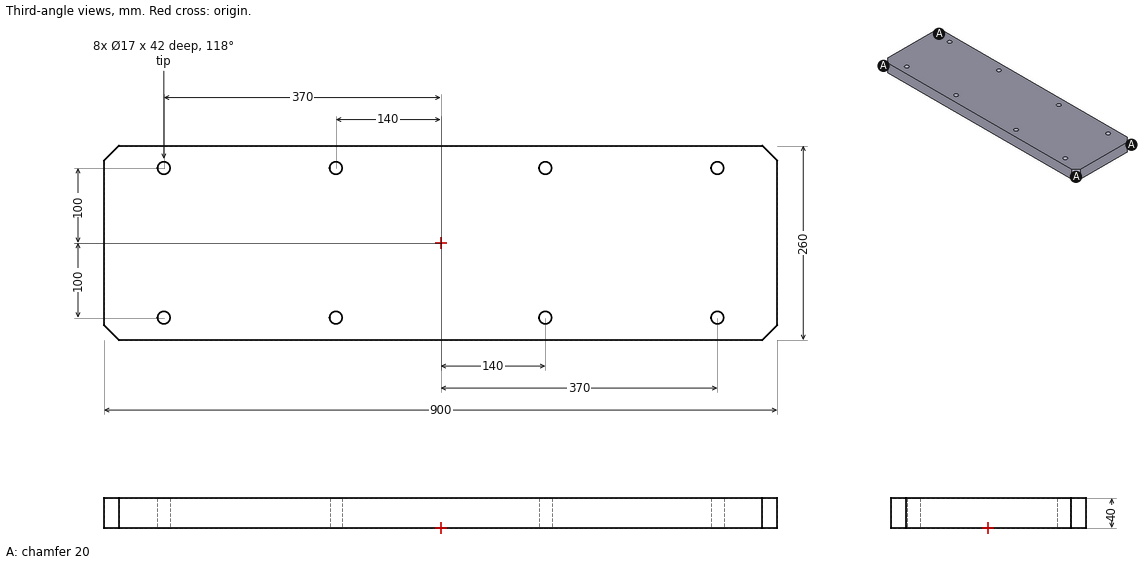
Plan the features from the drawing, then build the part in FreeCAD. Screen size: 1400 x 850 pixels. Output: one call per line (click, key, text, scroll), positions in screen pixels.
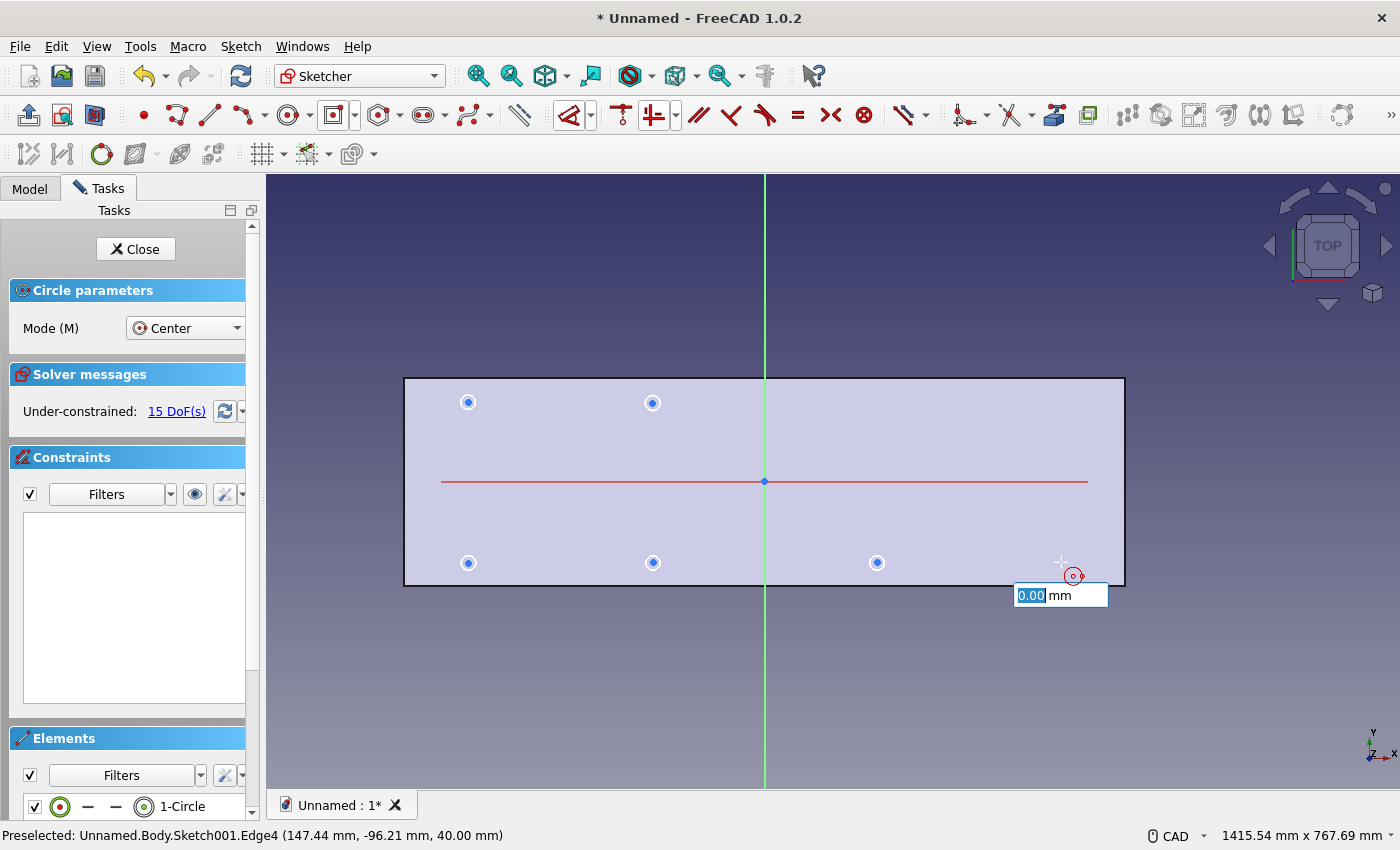
scroll(1066, 557, up, 5)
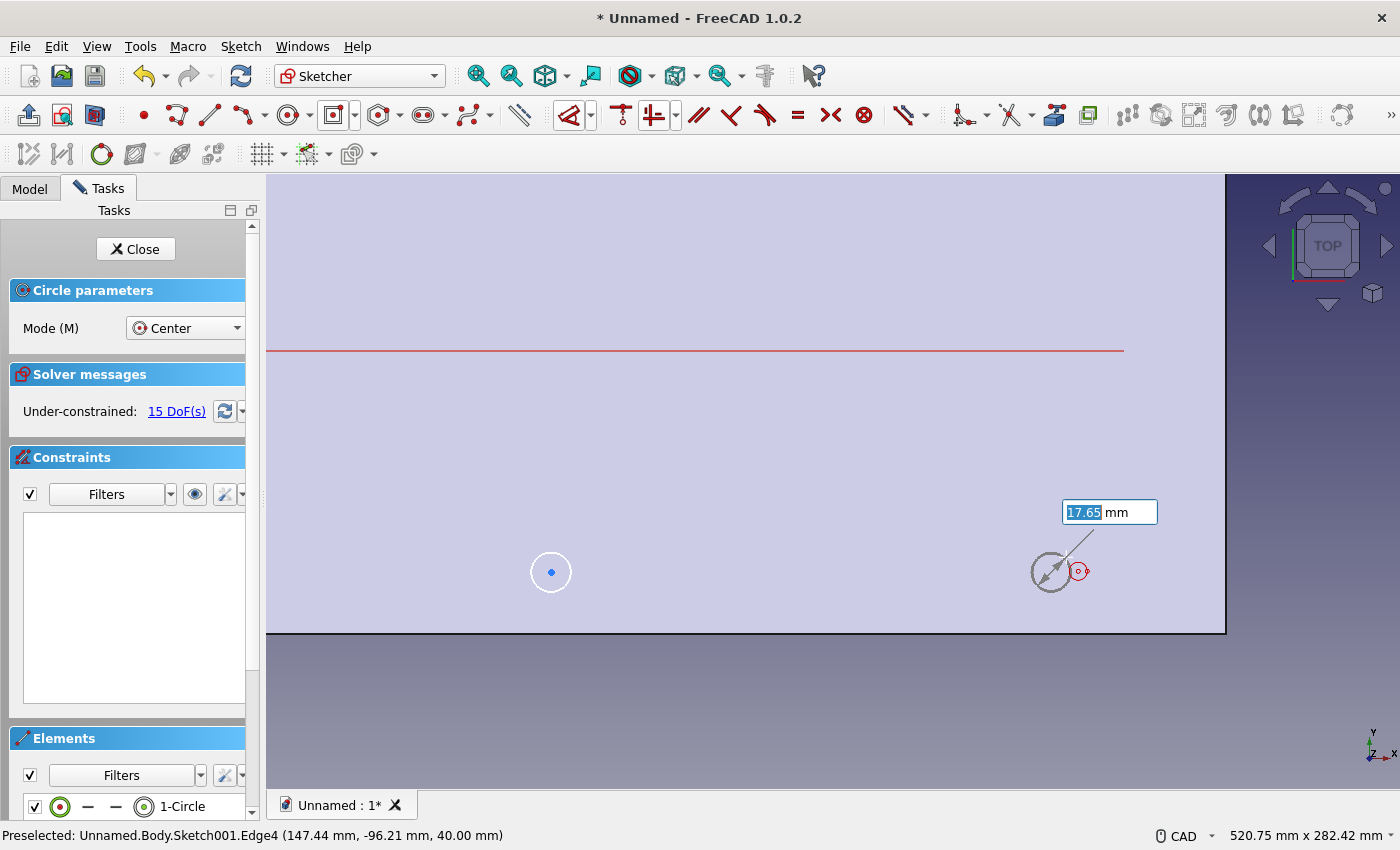
click(1065, 556)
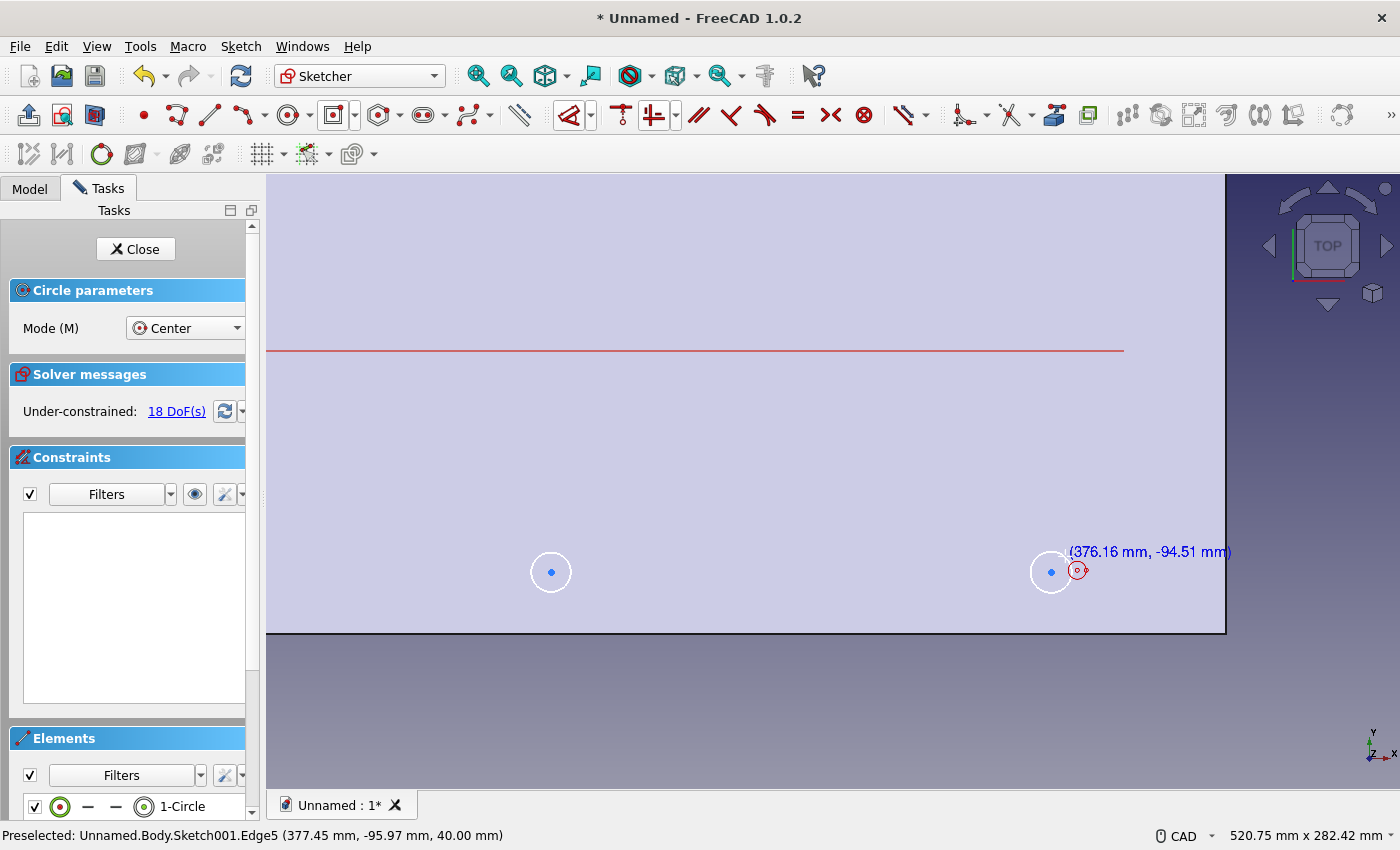
scroll(1066, 557, down, 5)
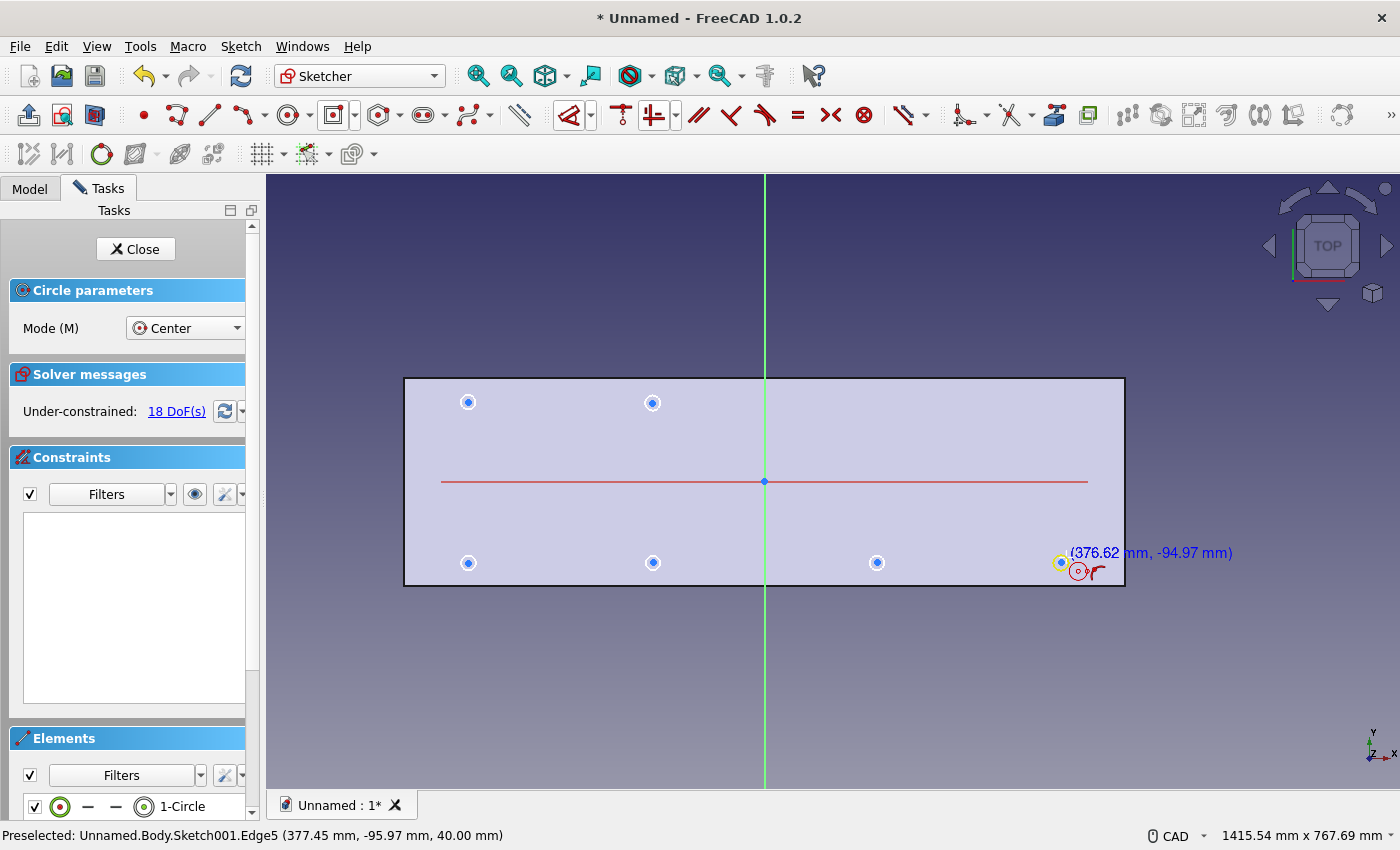
scroll(877, 402, up, 7)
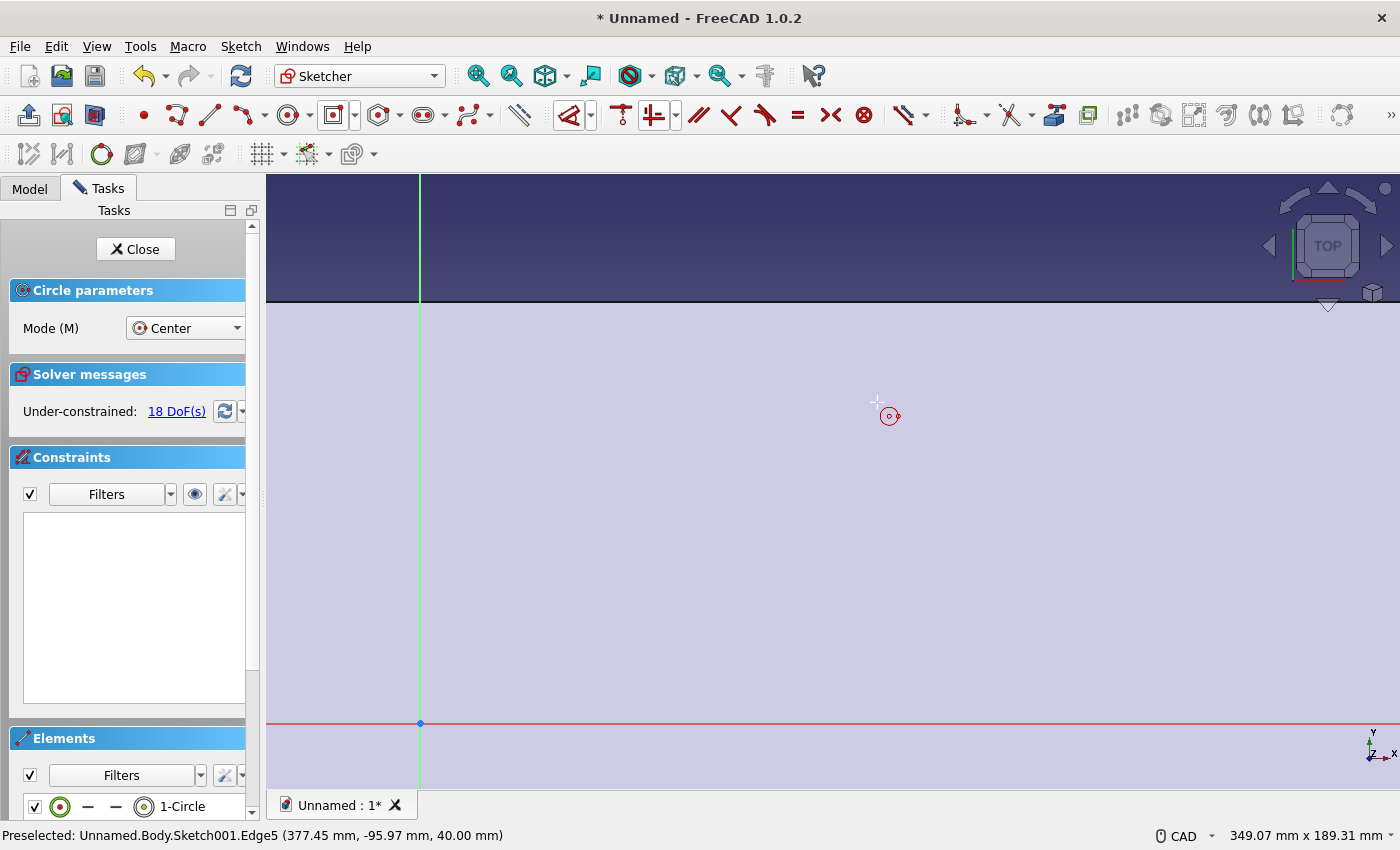
scroll(877, 402, down, 7)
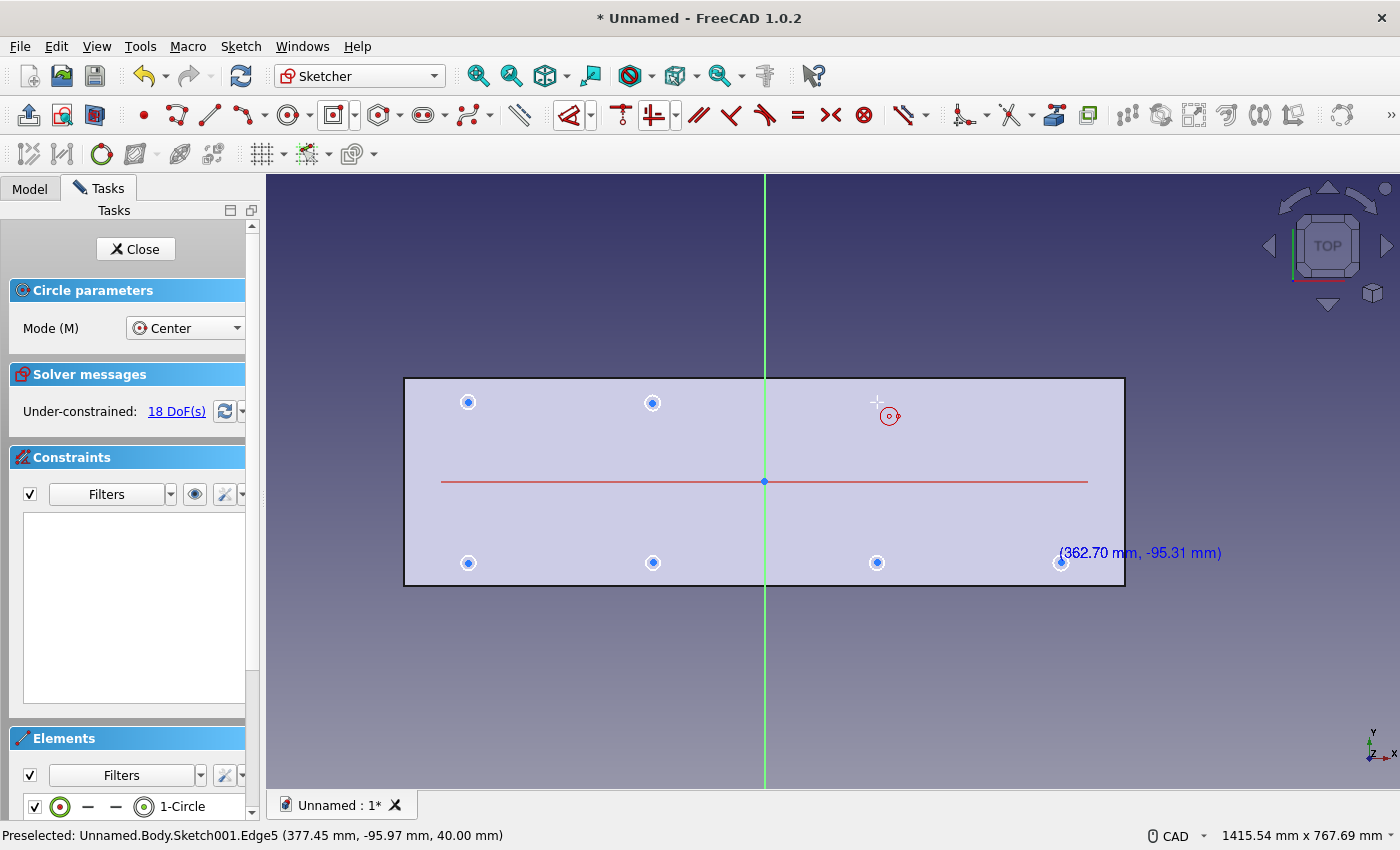
click(877, 402)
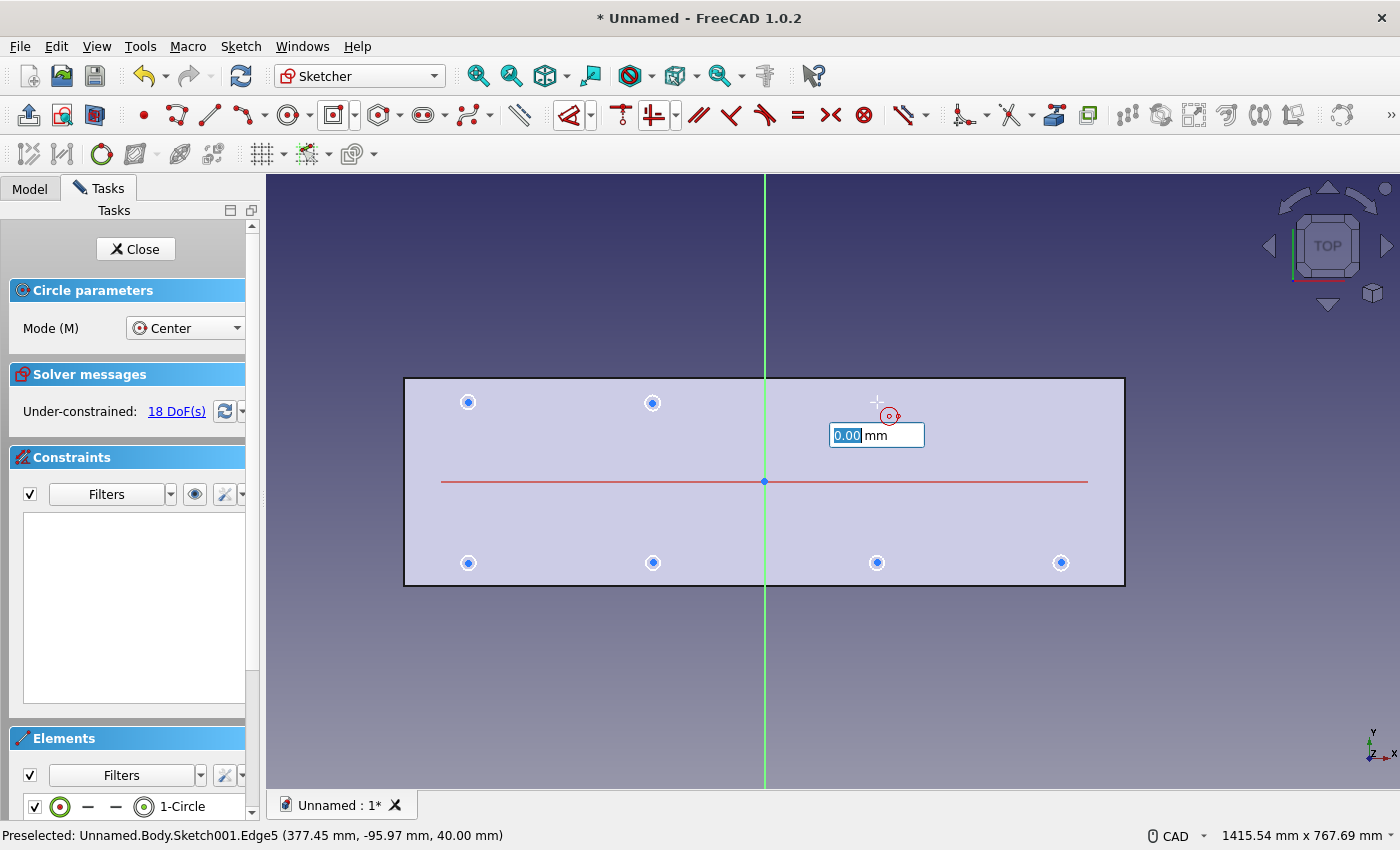
scroll(882, 397, up, 5)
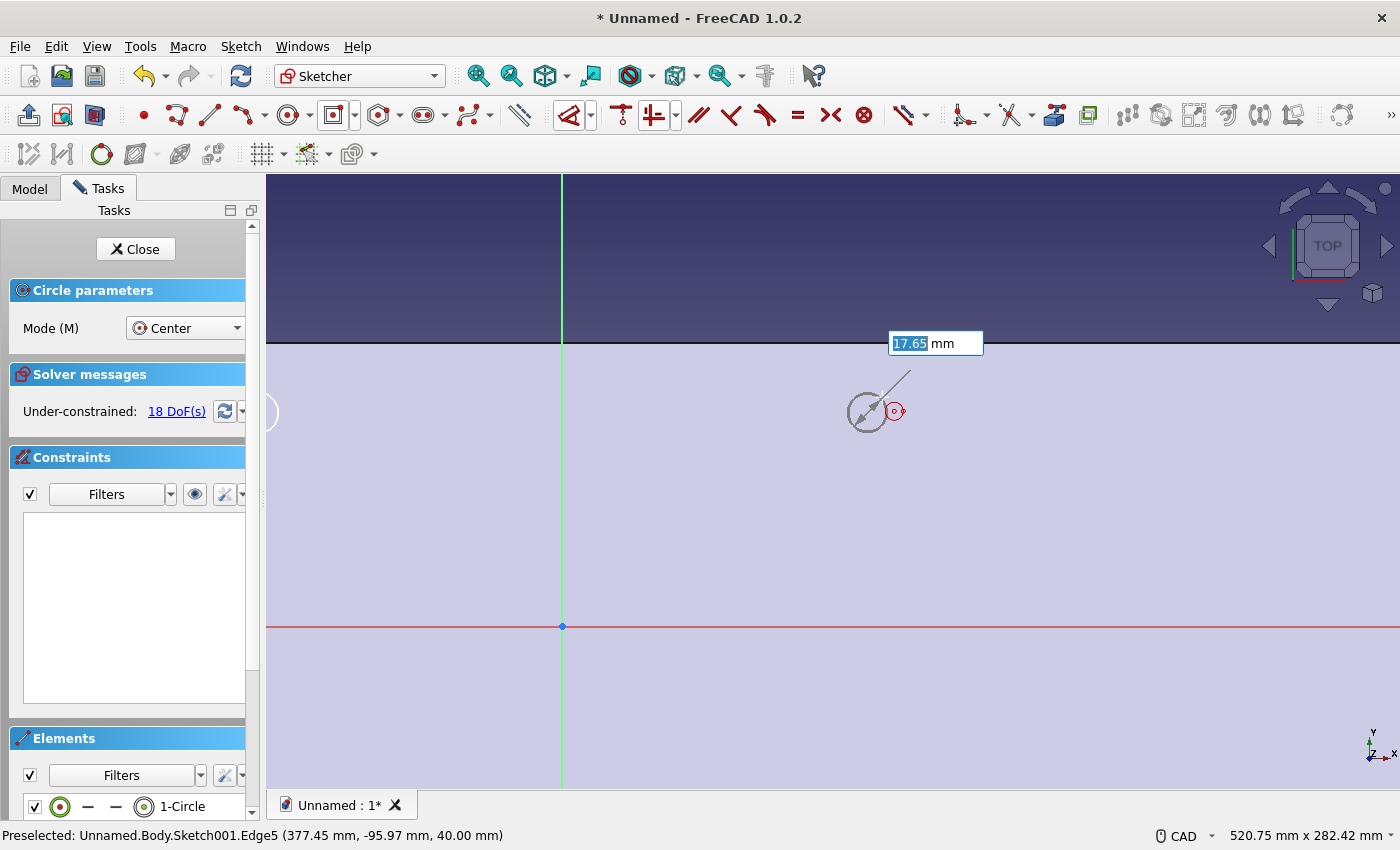
click(880, 396)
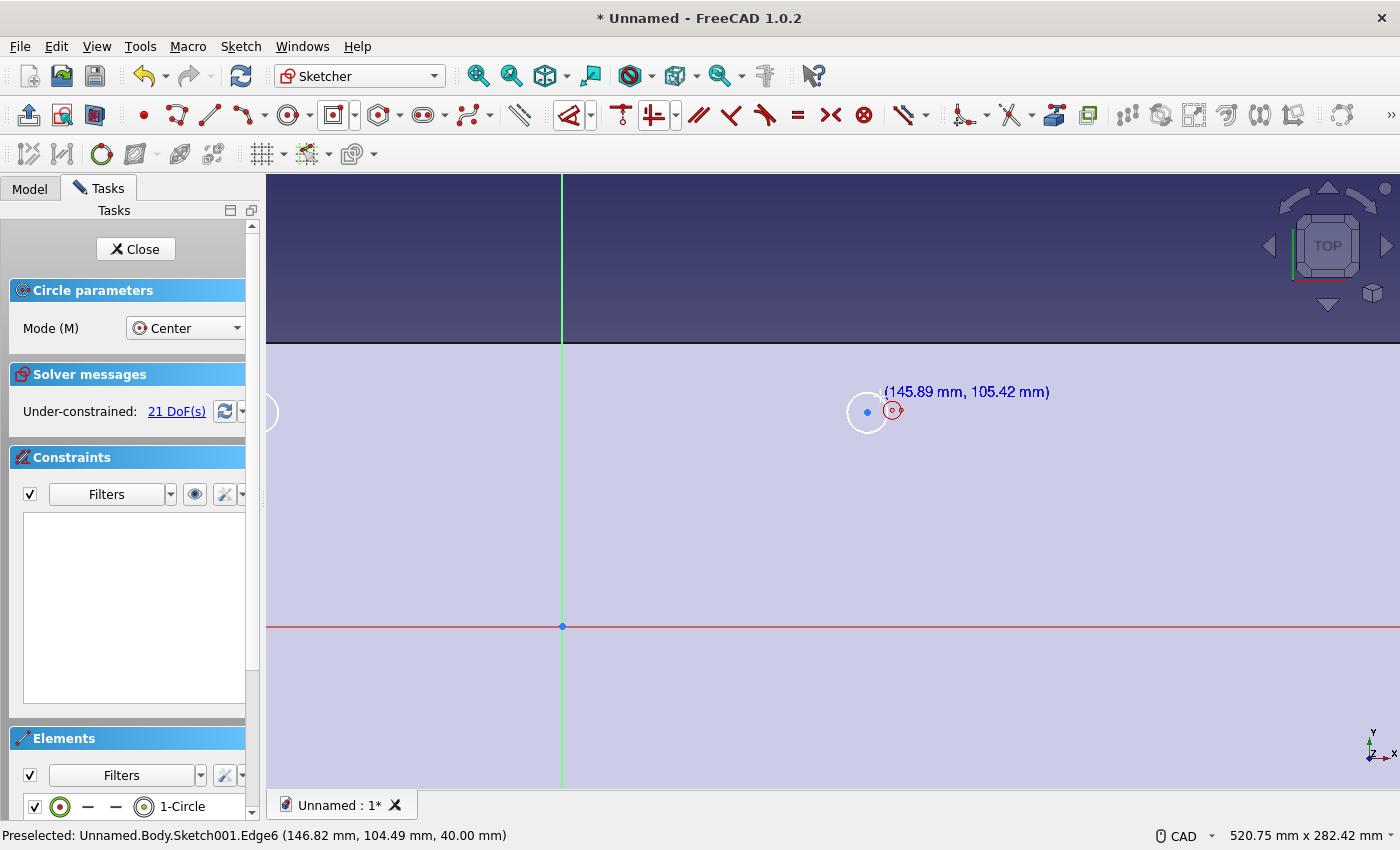
scroll(882, 397, down, 5)